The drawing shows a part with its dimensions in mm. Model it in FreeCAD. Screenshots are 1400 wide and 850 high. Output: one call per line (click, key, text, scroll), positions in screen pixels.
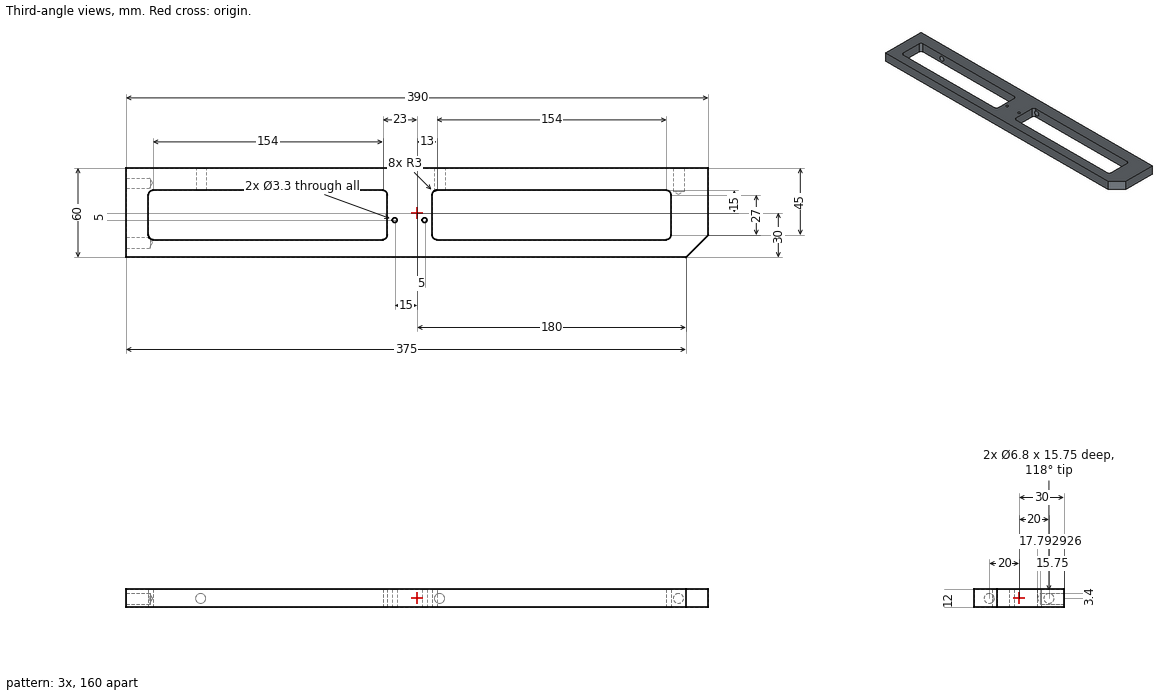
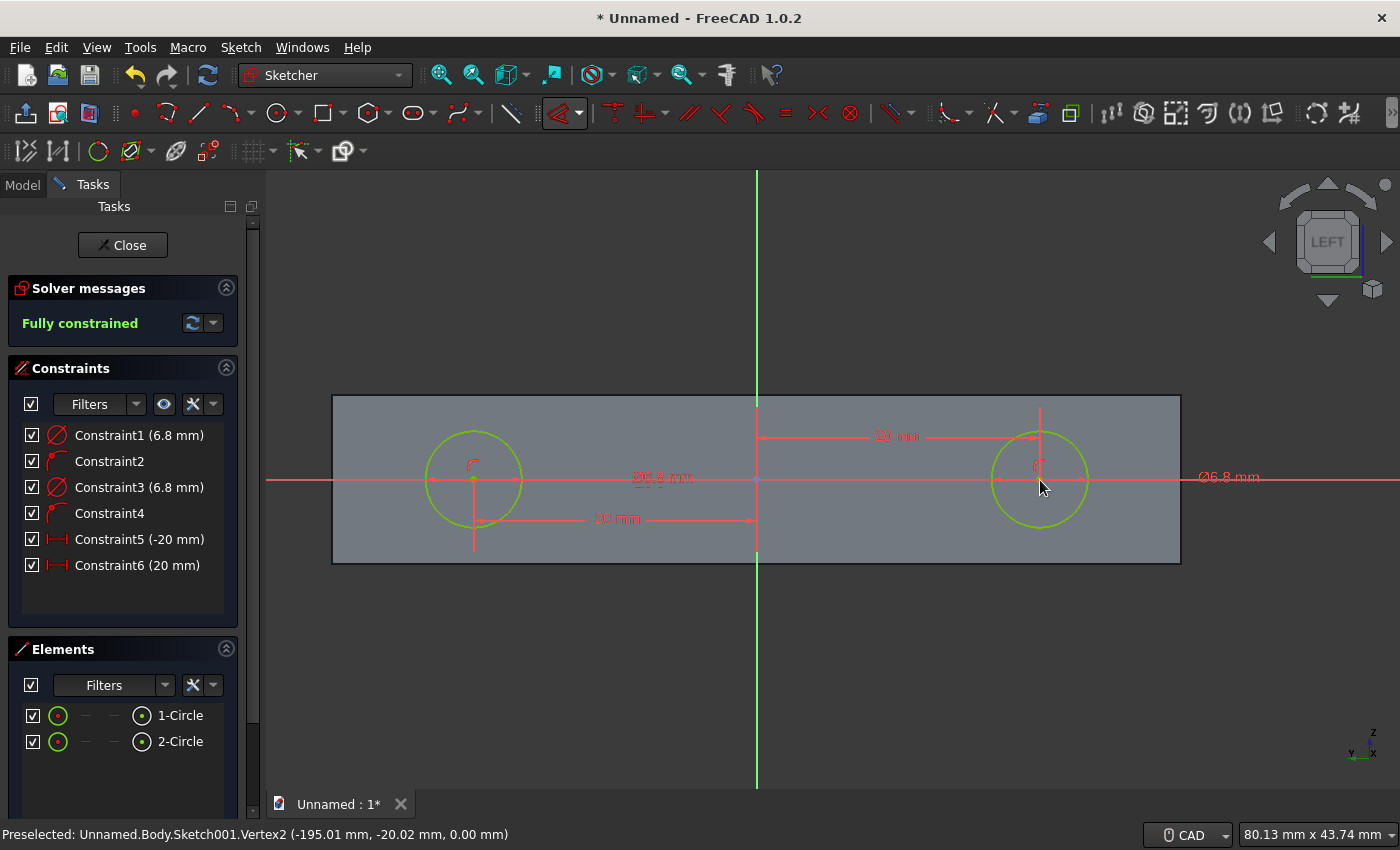
click(123, 245)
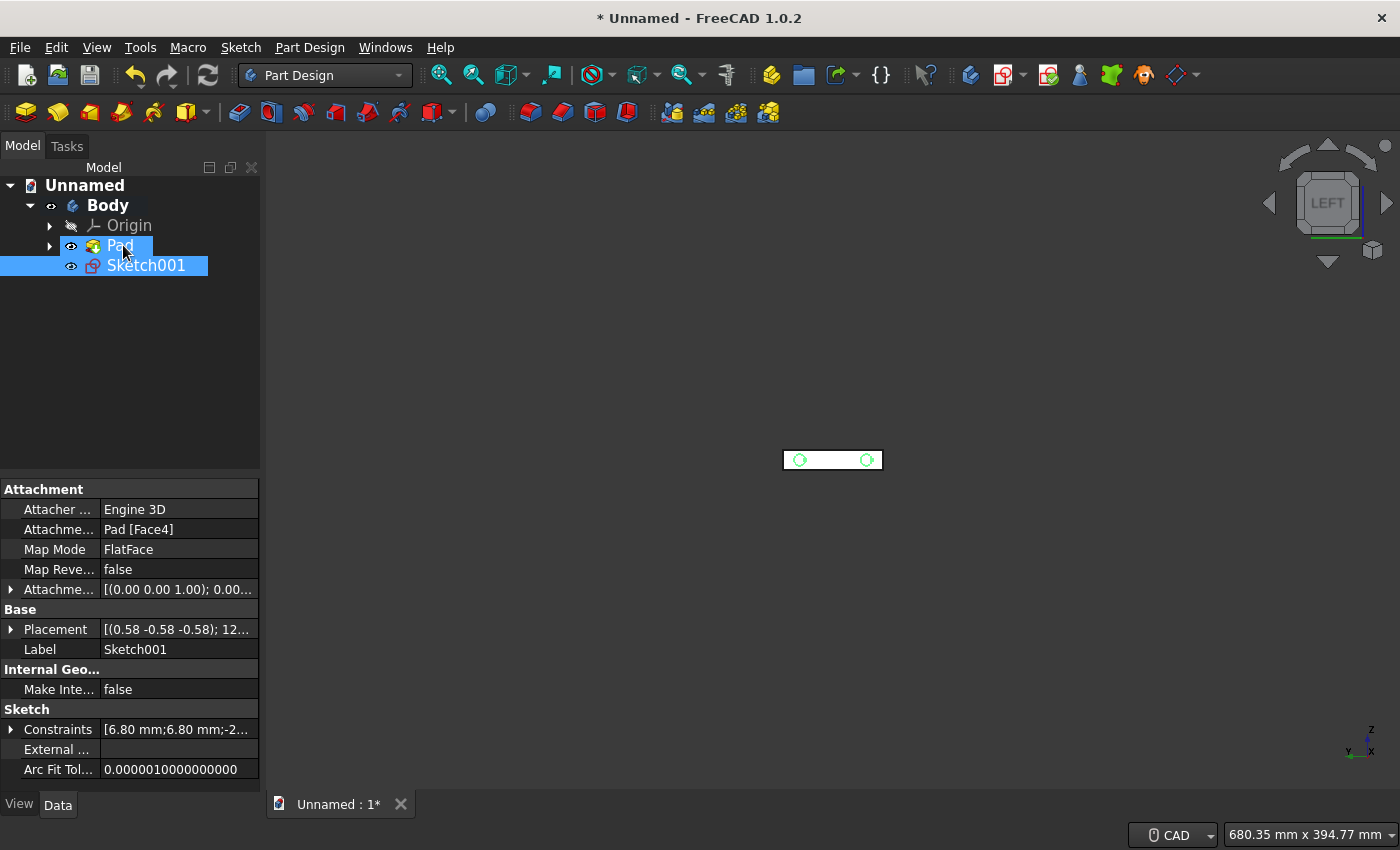
click(272, 112)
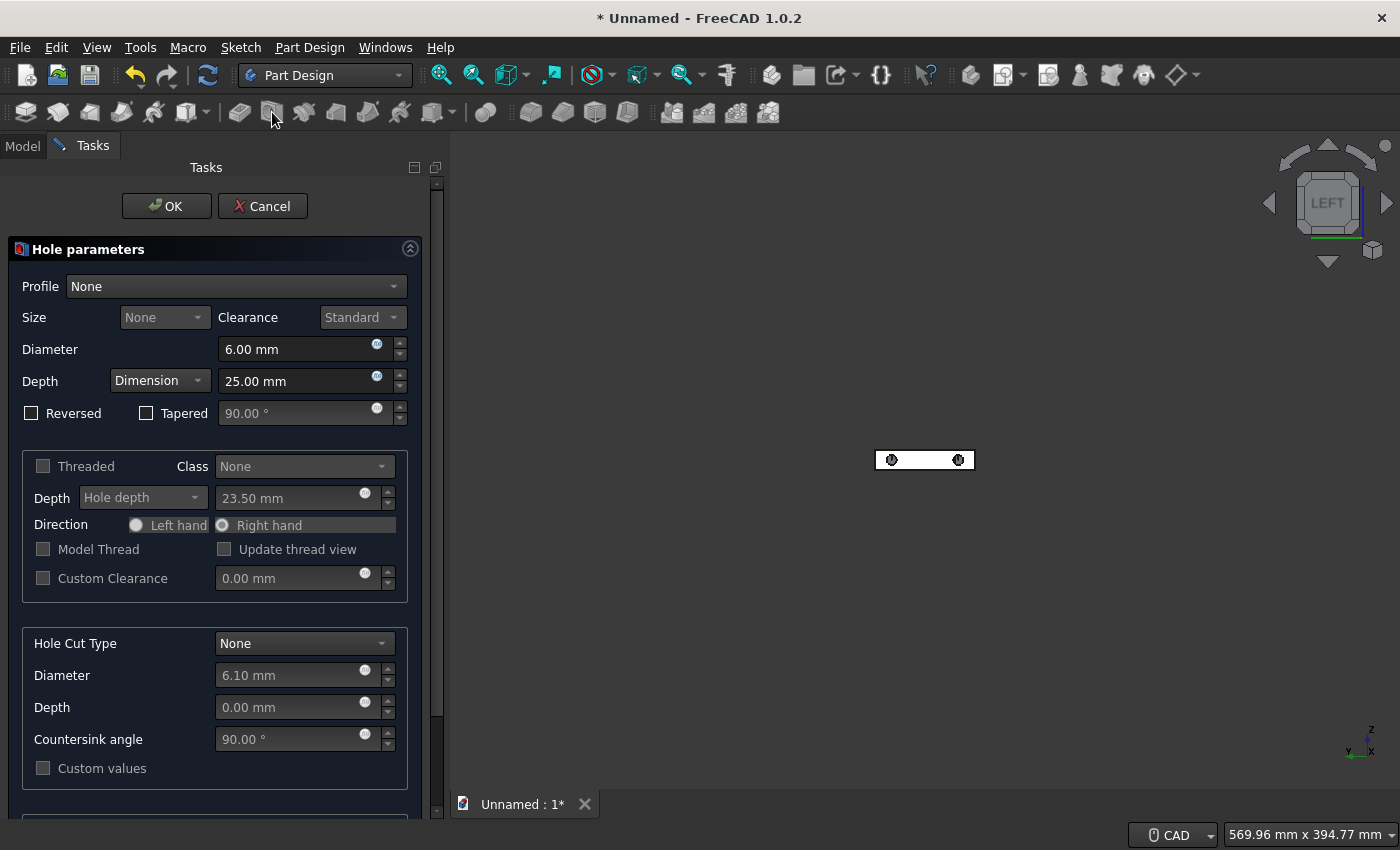
triple_click(305, 349)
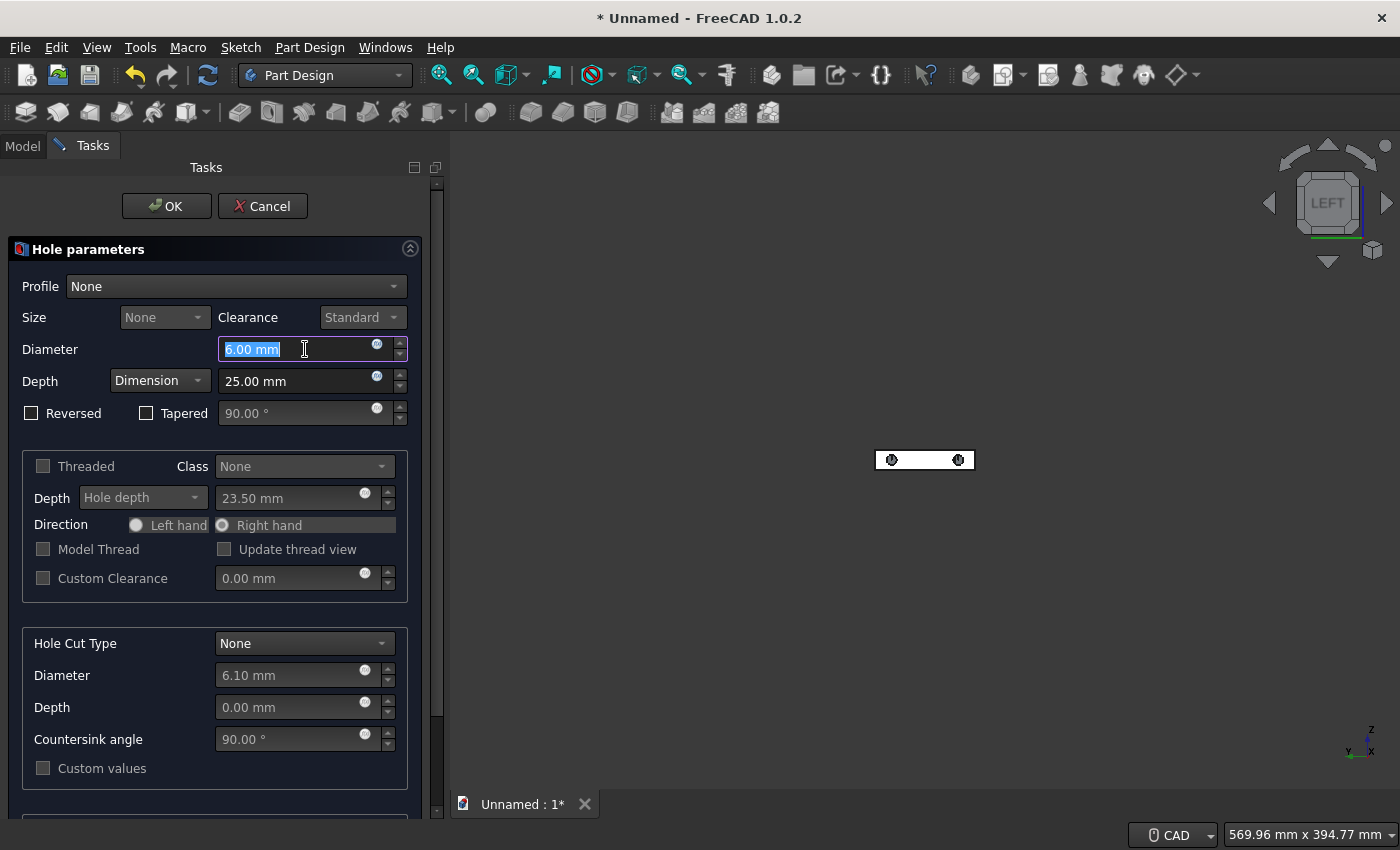
text(6.8)
key(Tab)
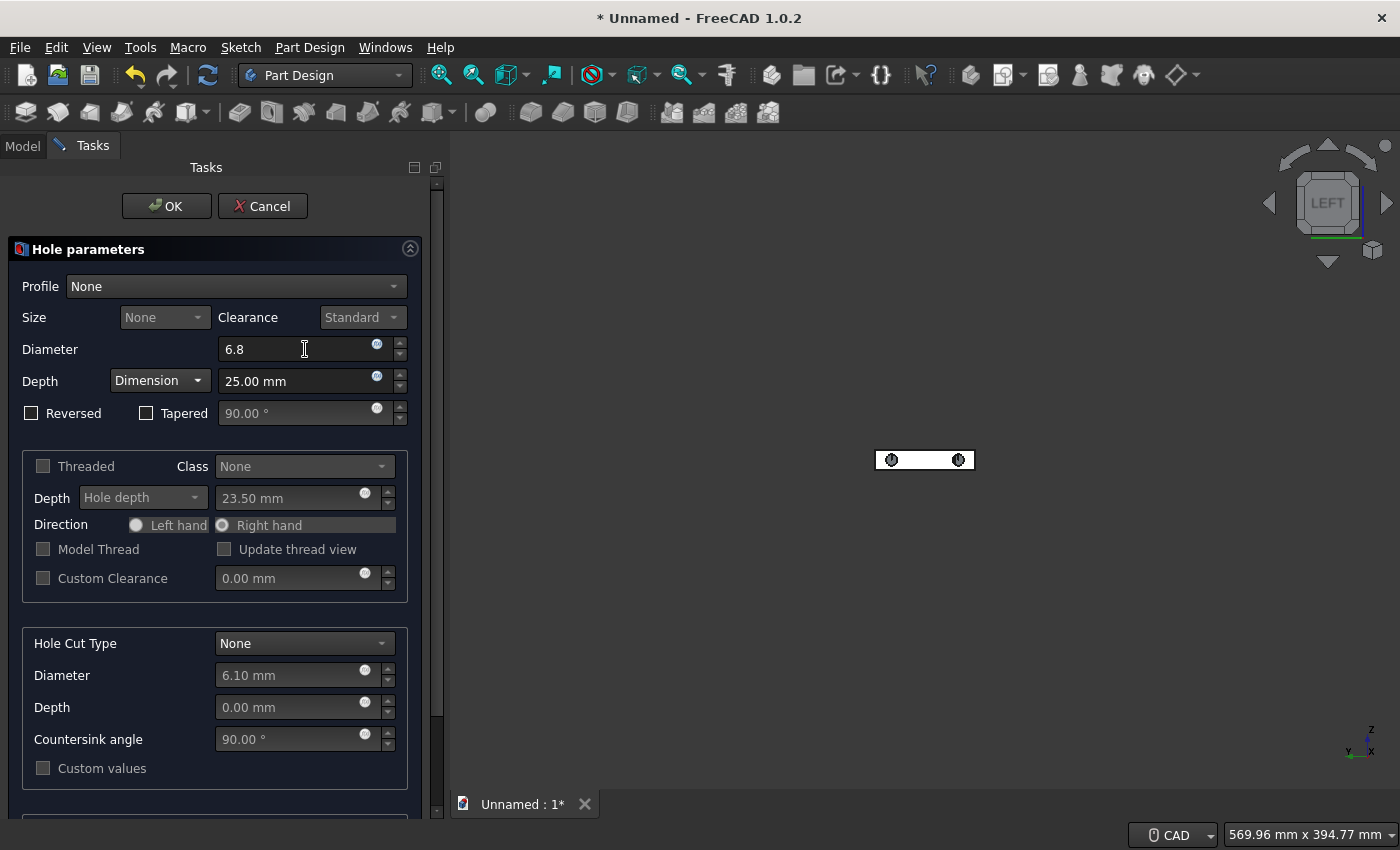
triple_click(305, 381)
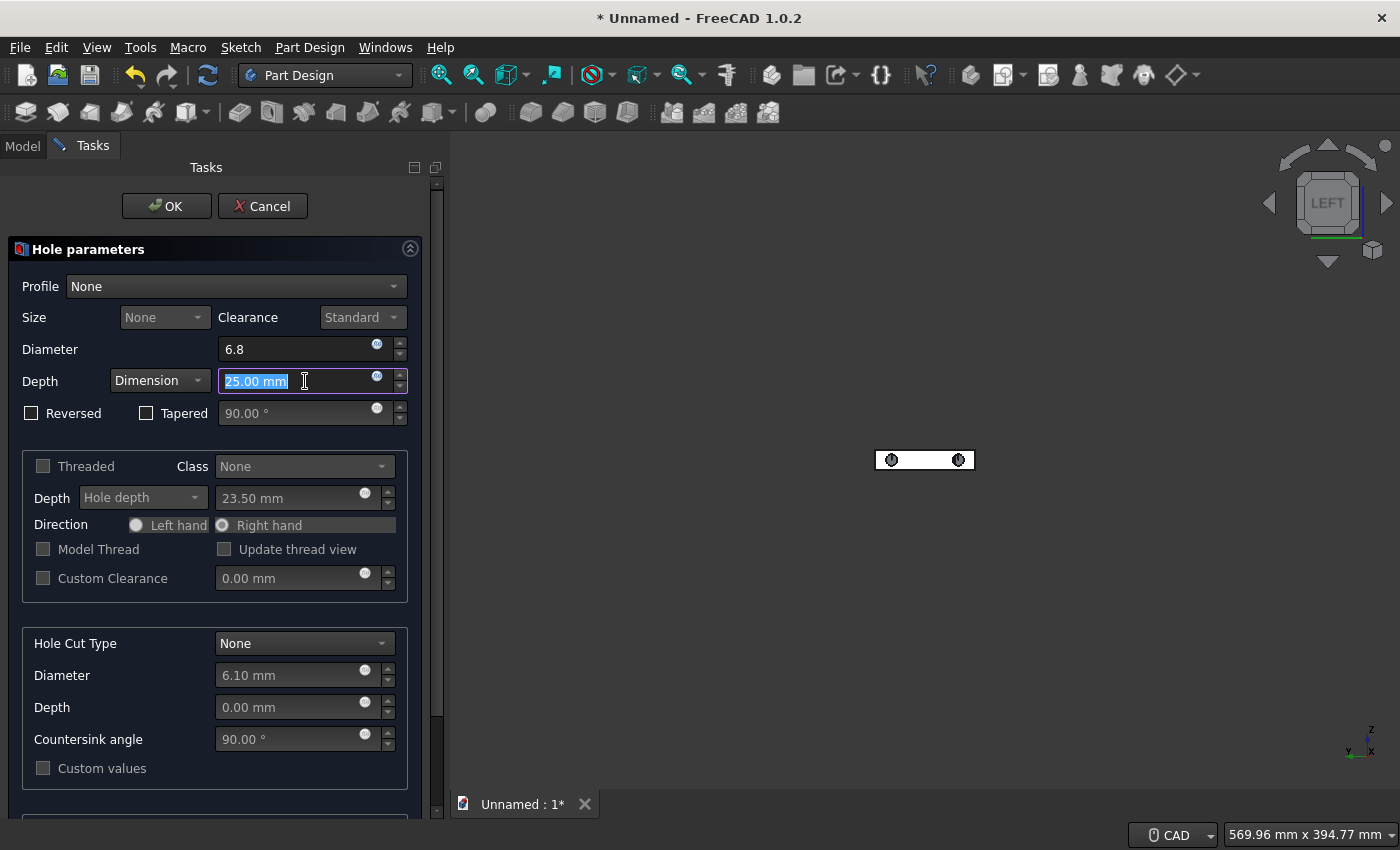
text(15.75)
key(Tab)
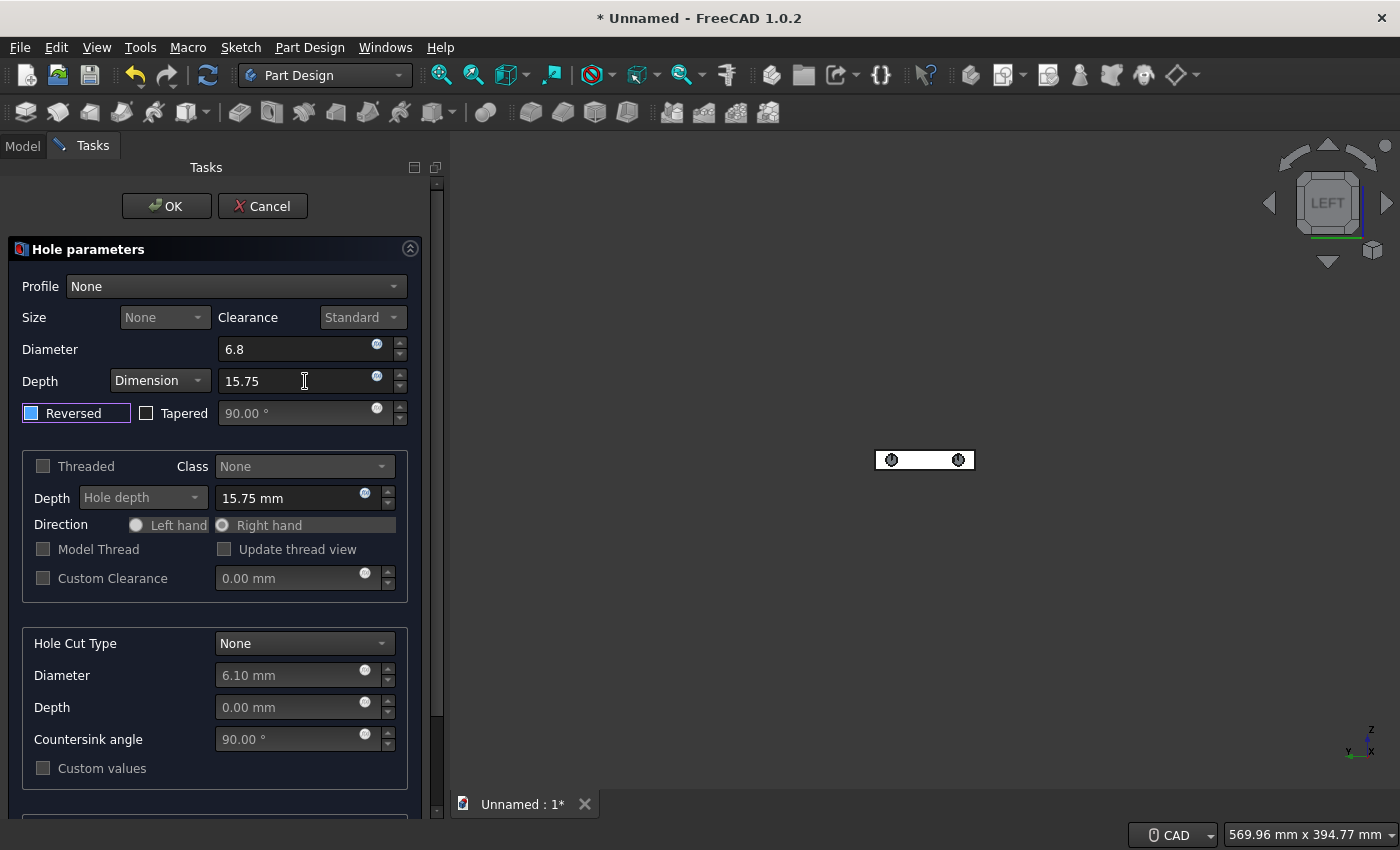
click(167, 206)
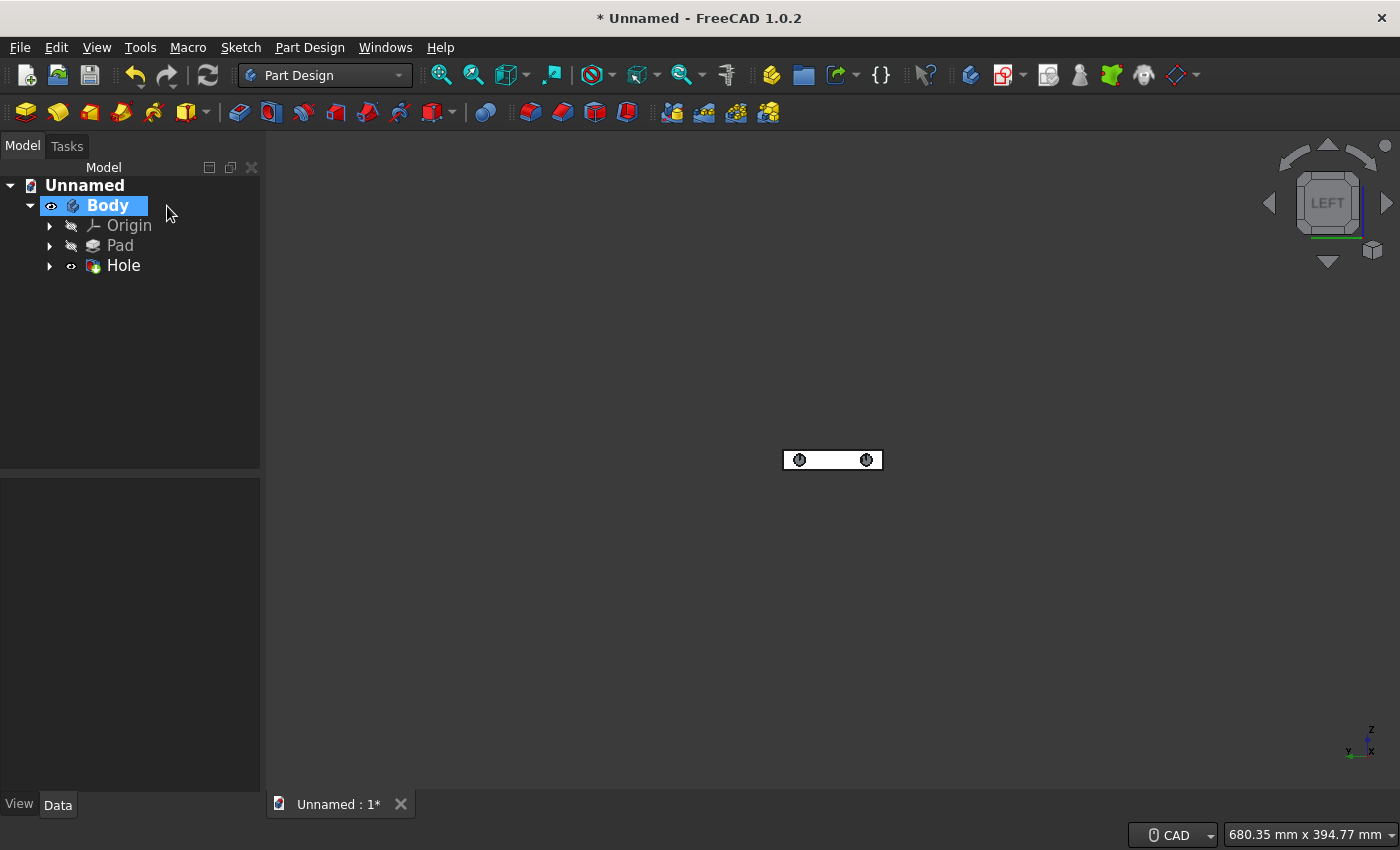
key(v)
key(f)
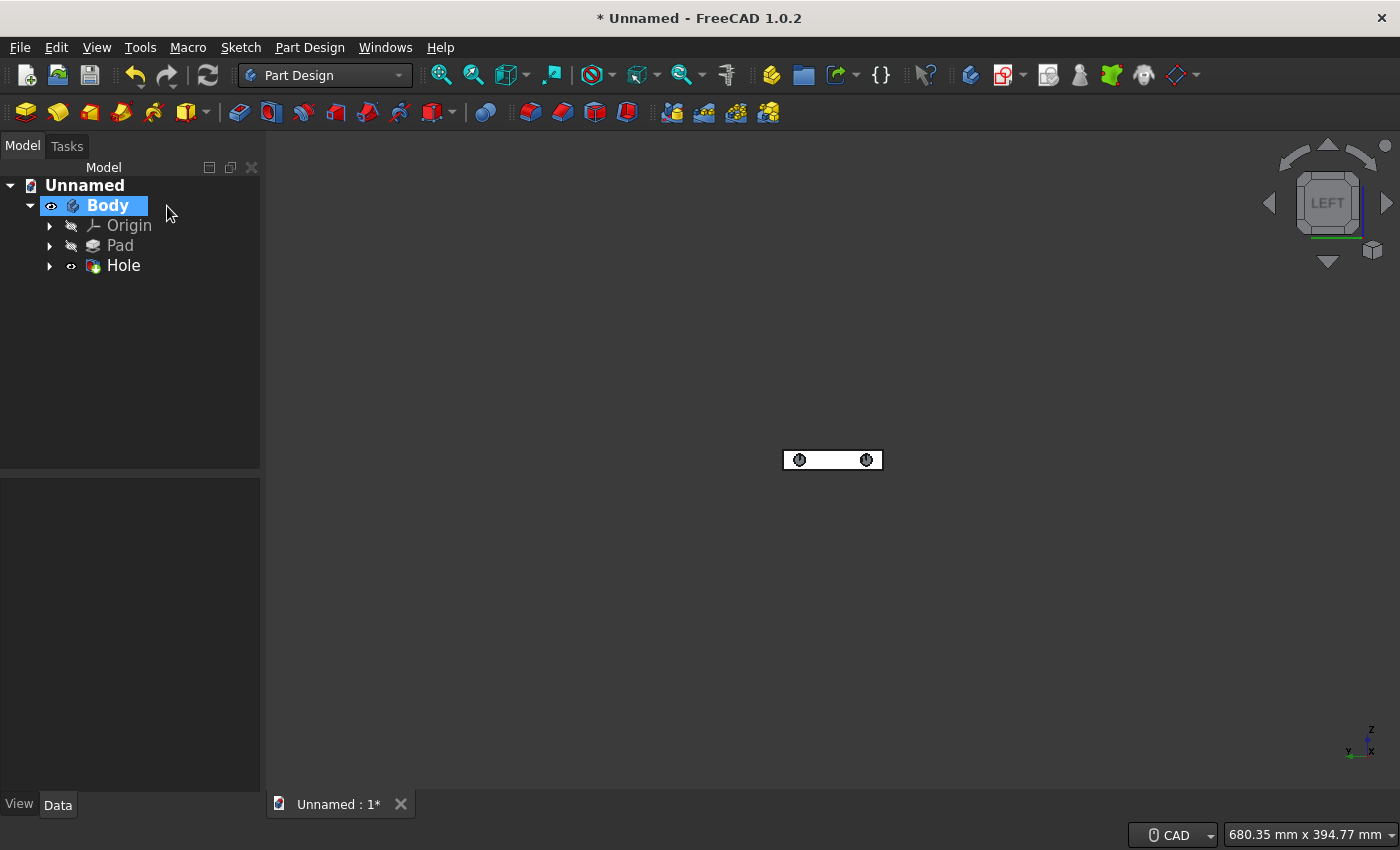
key(0)